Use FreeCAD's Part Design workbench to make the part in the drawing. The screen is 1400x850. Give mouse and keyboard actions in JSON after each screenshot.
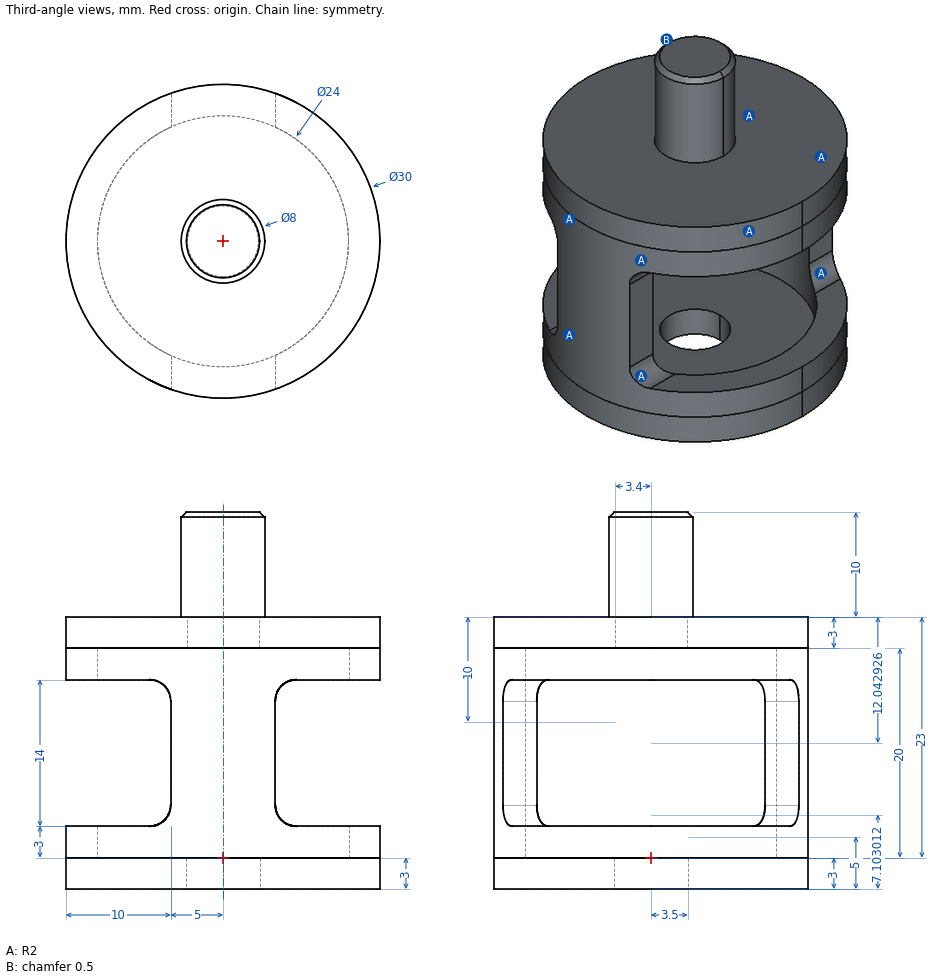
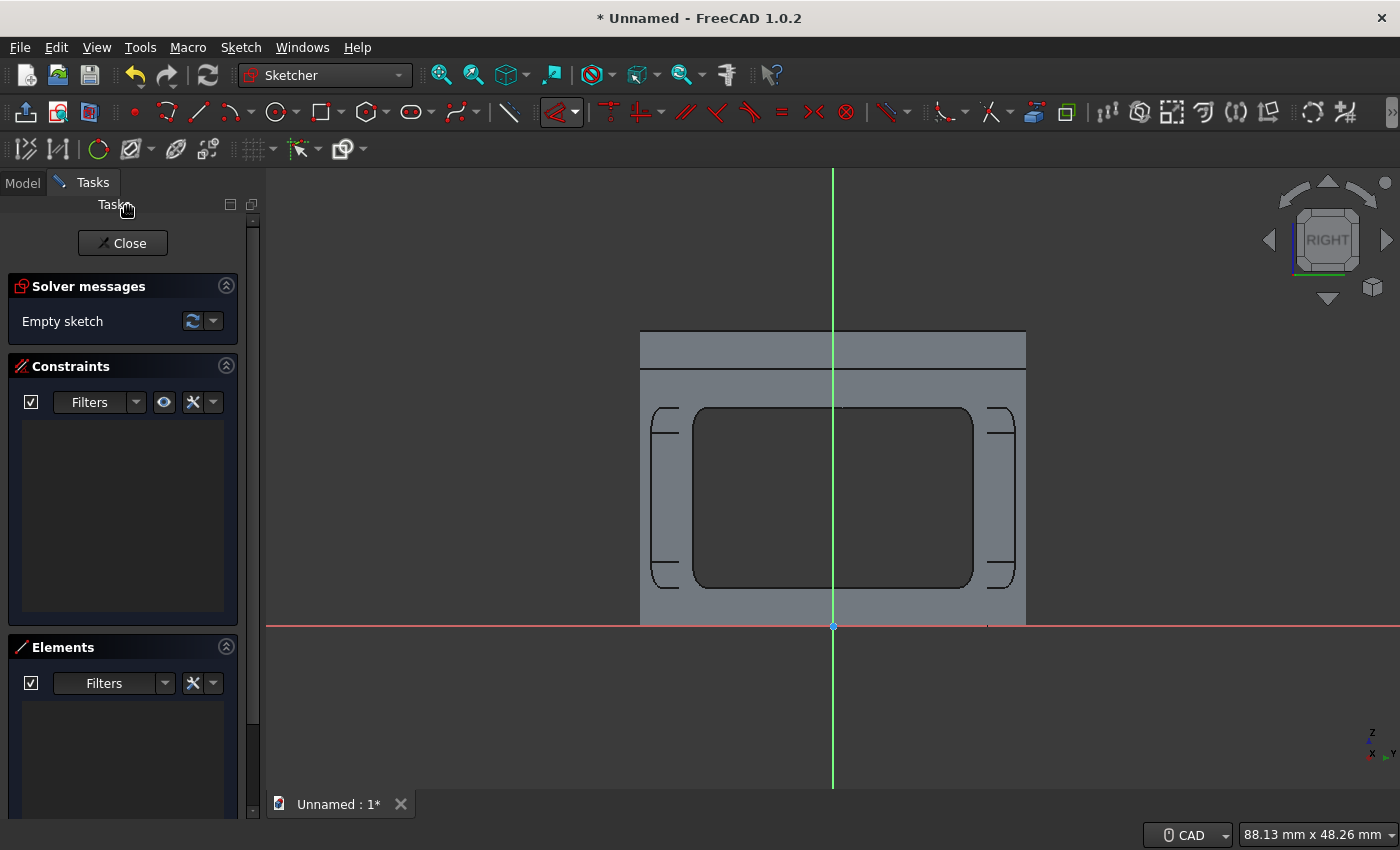
{"action": "left_click", "coordinate": [833, 485]}
{"action": "left_click", "coordinate": [824, 331]}
{"action": "left_click", "coordinate": [789, 331]}
{"action": "left_click", "coordinate": [789, 459]}
{"action": "left_click", "coordinate": [833, 486]}
{"action": "key", "text": "Escape"}
{"action": "key", "text": "Escape"}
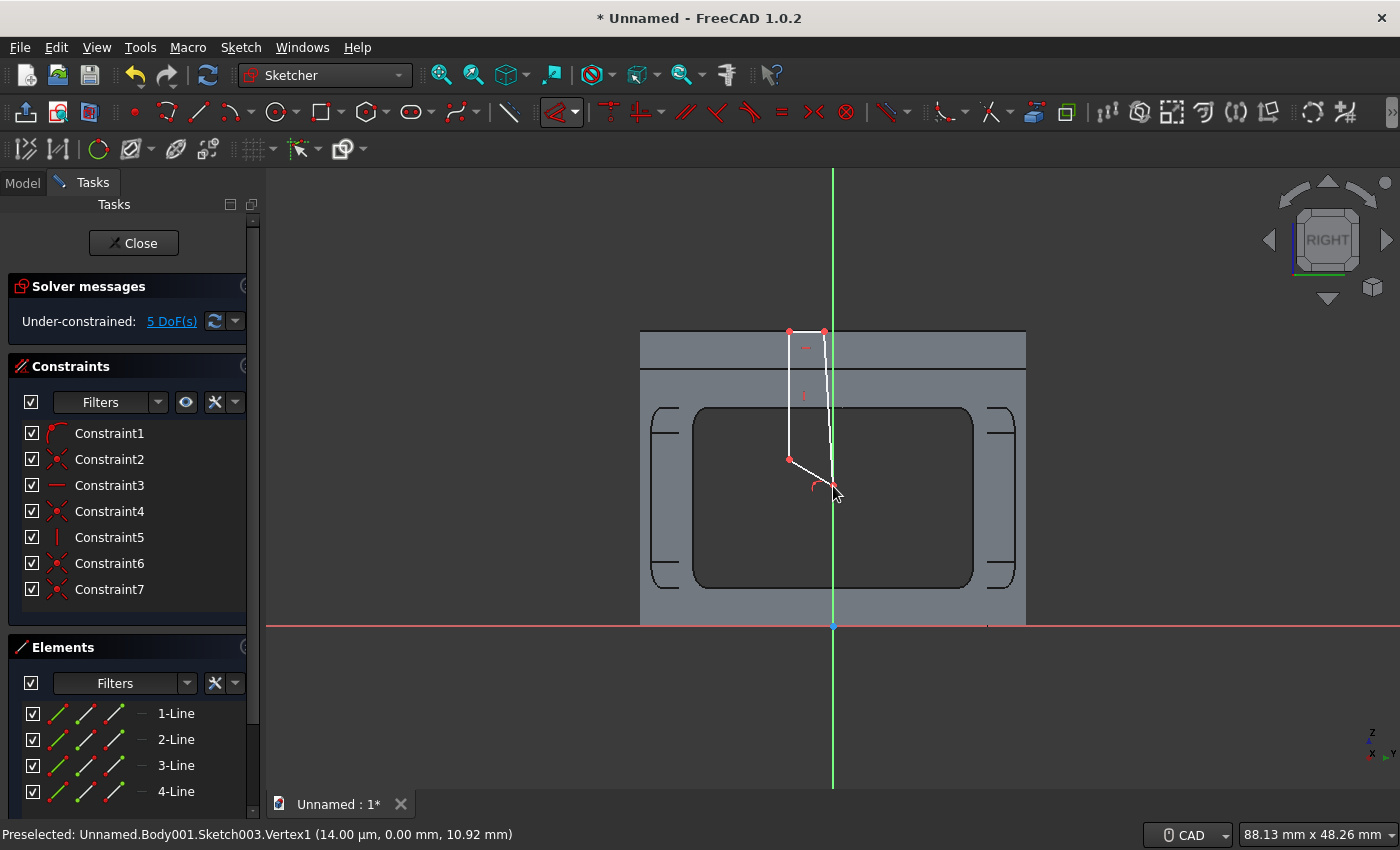
{"action": "left_click", "coordinate": [830, 440]}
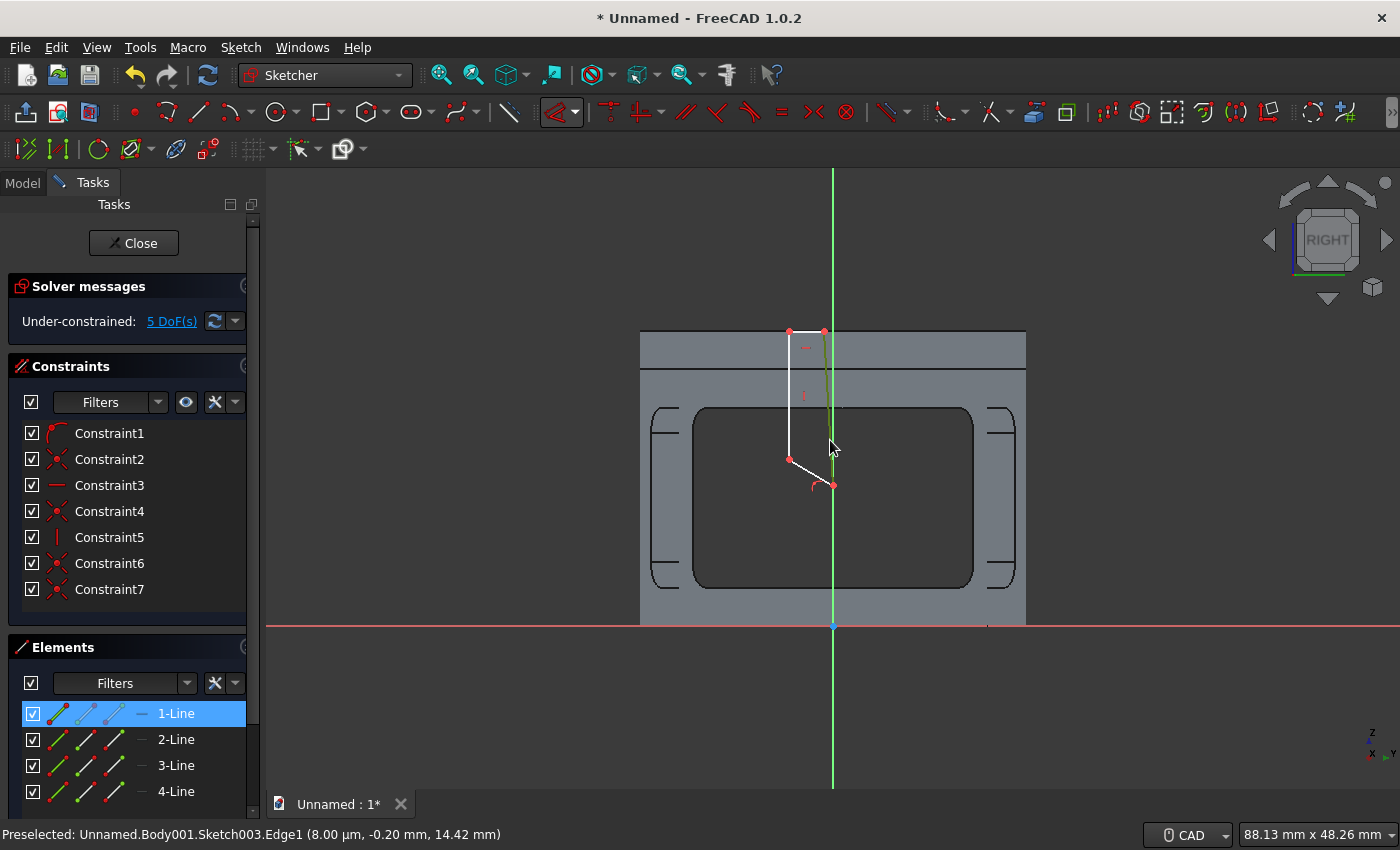
{"action": "key", "text": "v"}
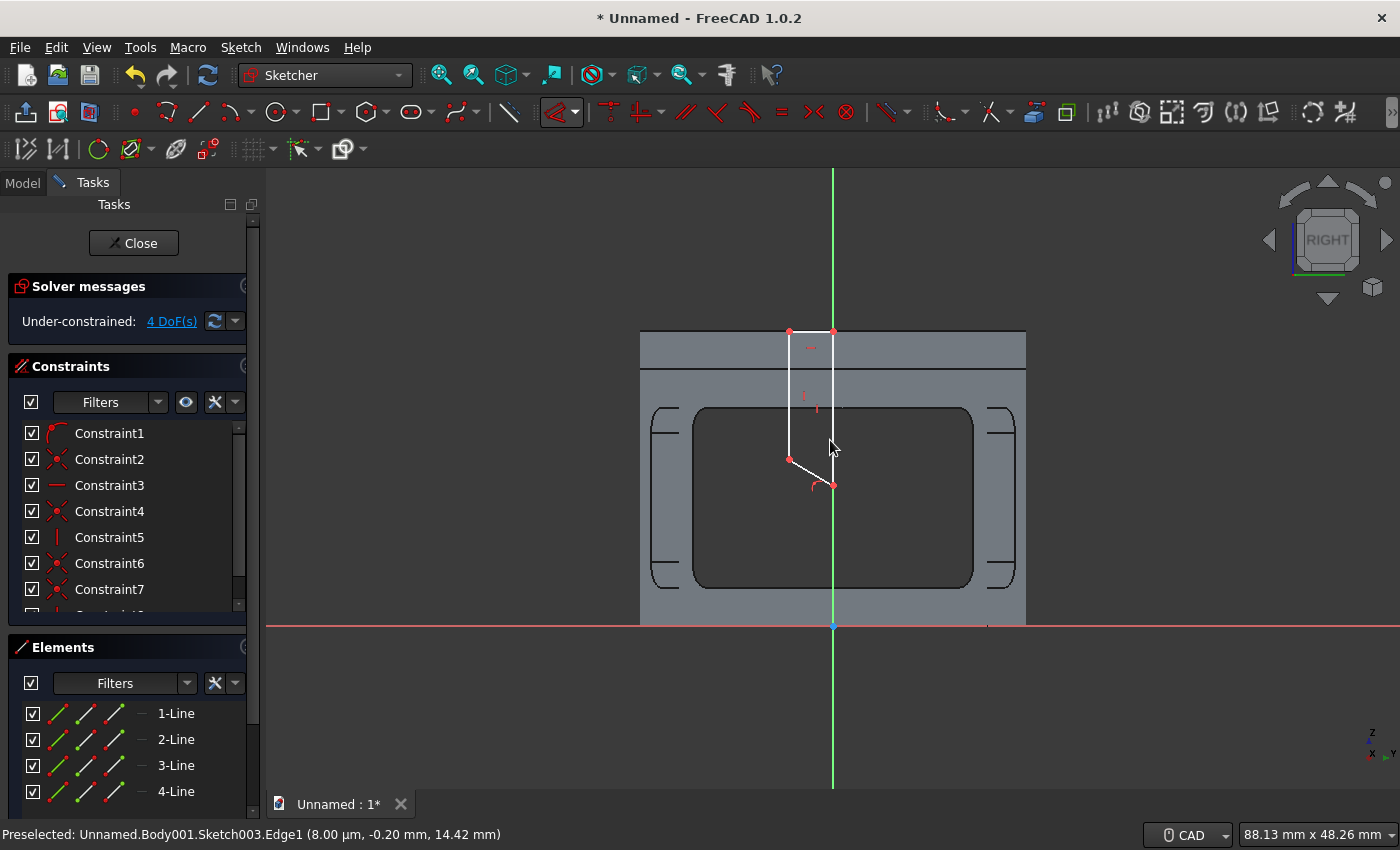
{"action": "left_click", "coordinate": [789, 370]}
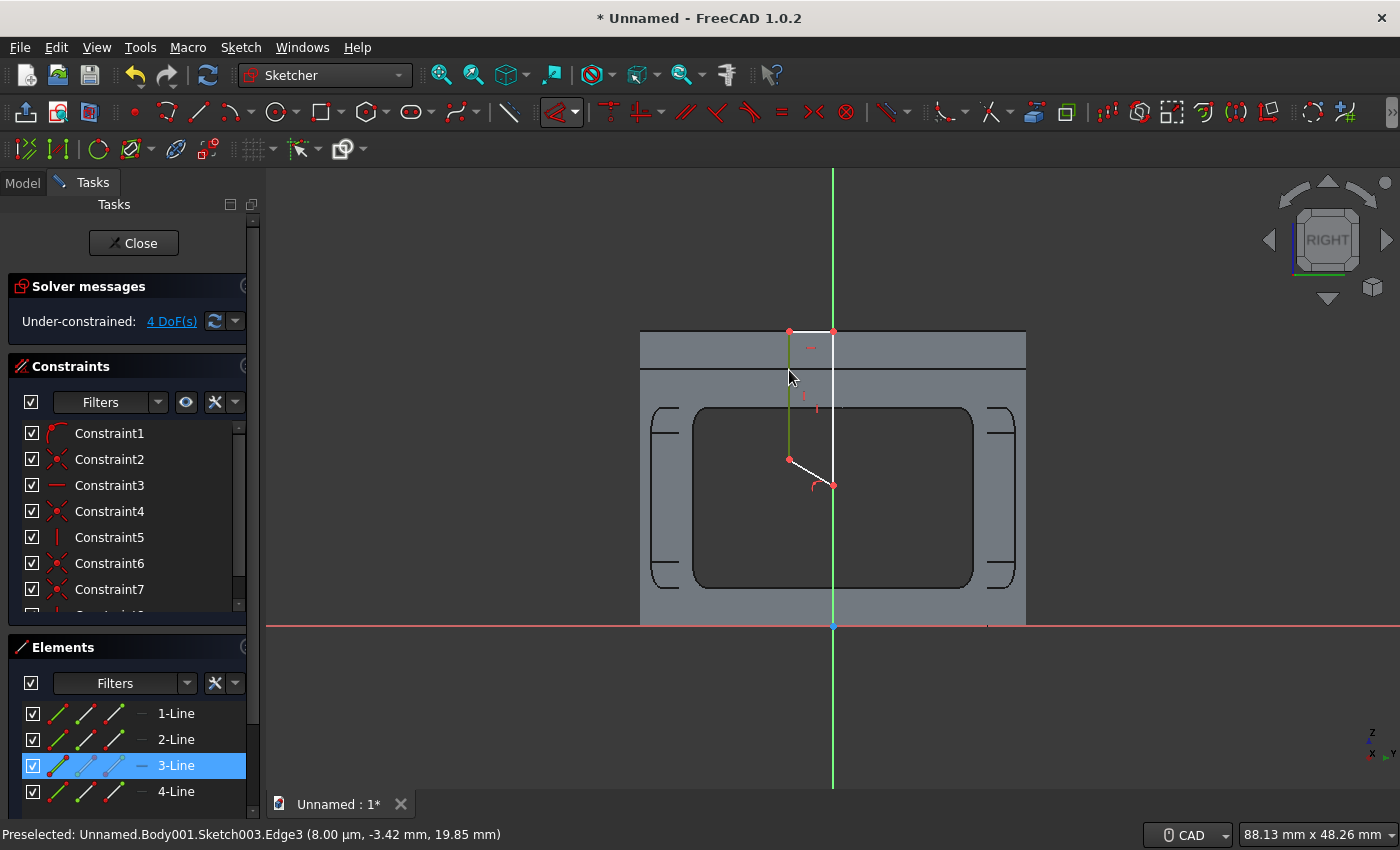
{"action": "key", "text": "i"}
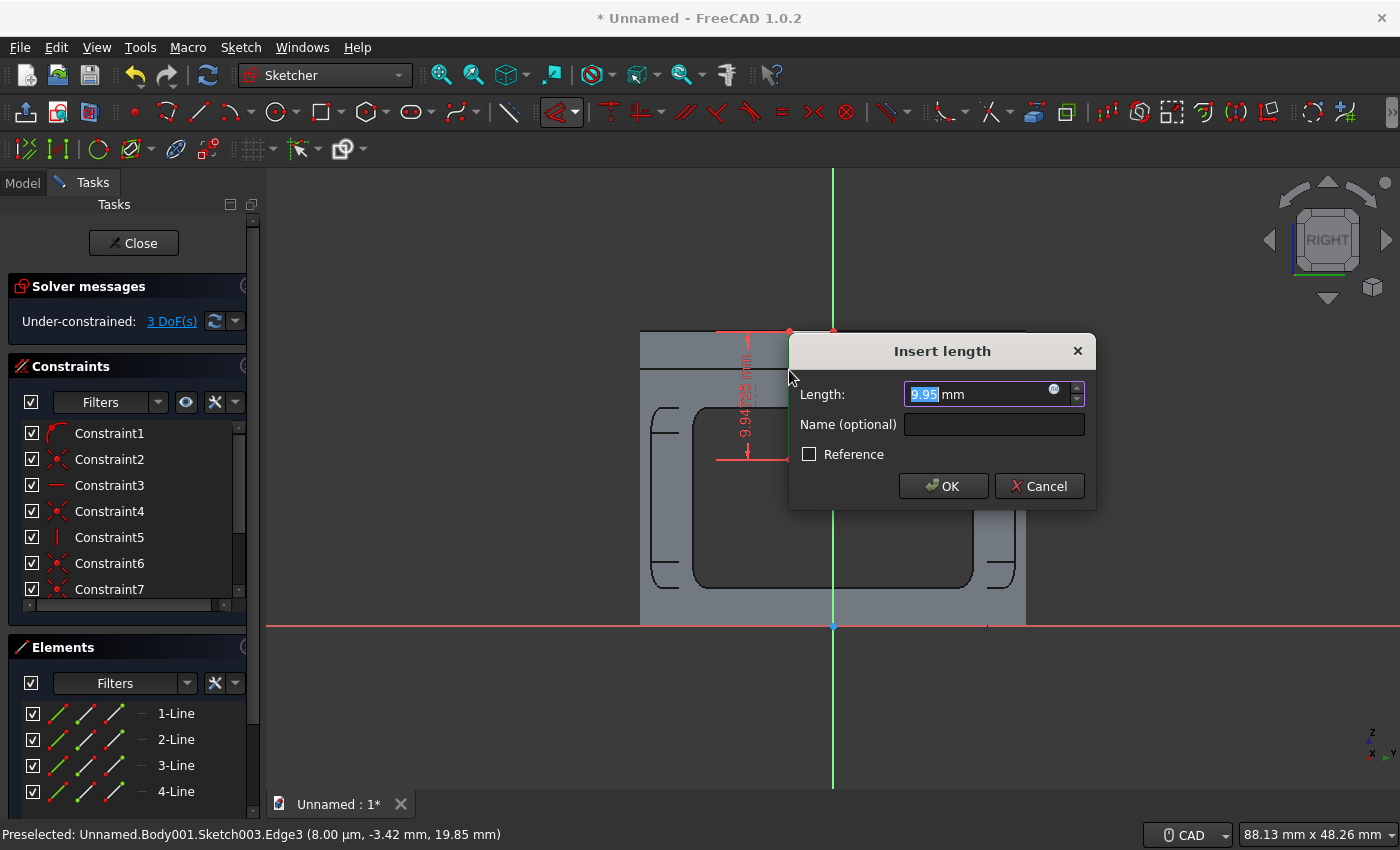
{"action": "type", "text": "10"}
{"action": "key", "text": "Return"}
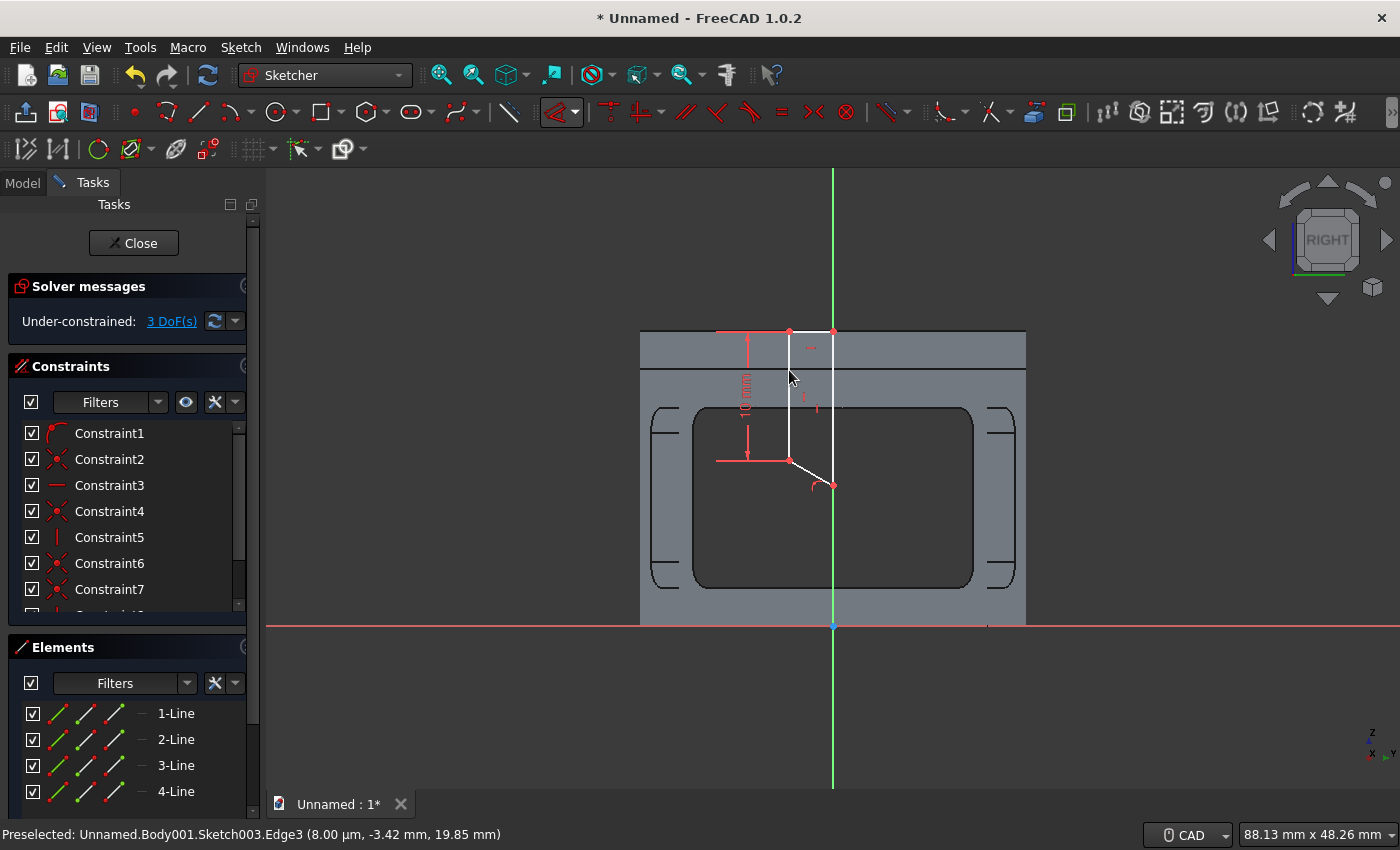
{"action": "left_click", "coordinate": [820, 332]}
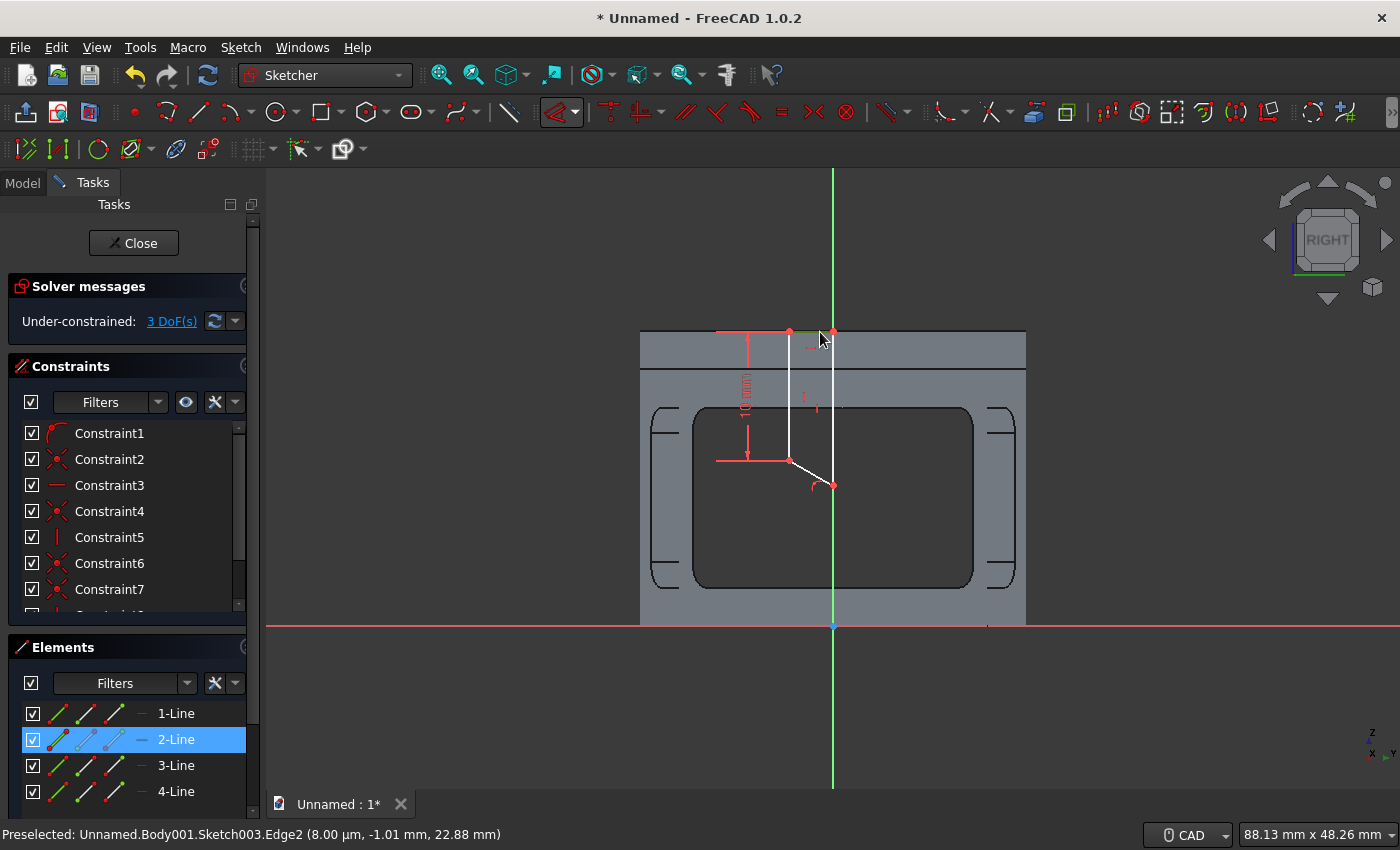
{"action": "key", "text": "l"}